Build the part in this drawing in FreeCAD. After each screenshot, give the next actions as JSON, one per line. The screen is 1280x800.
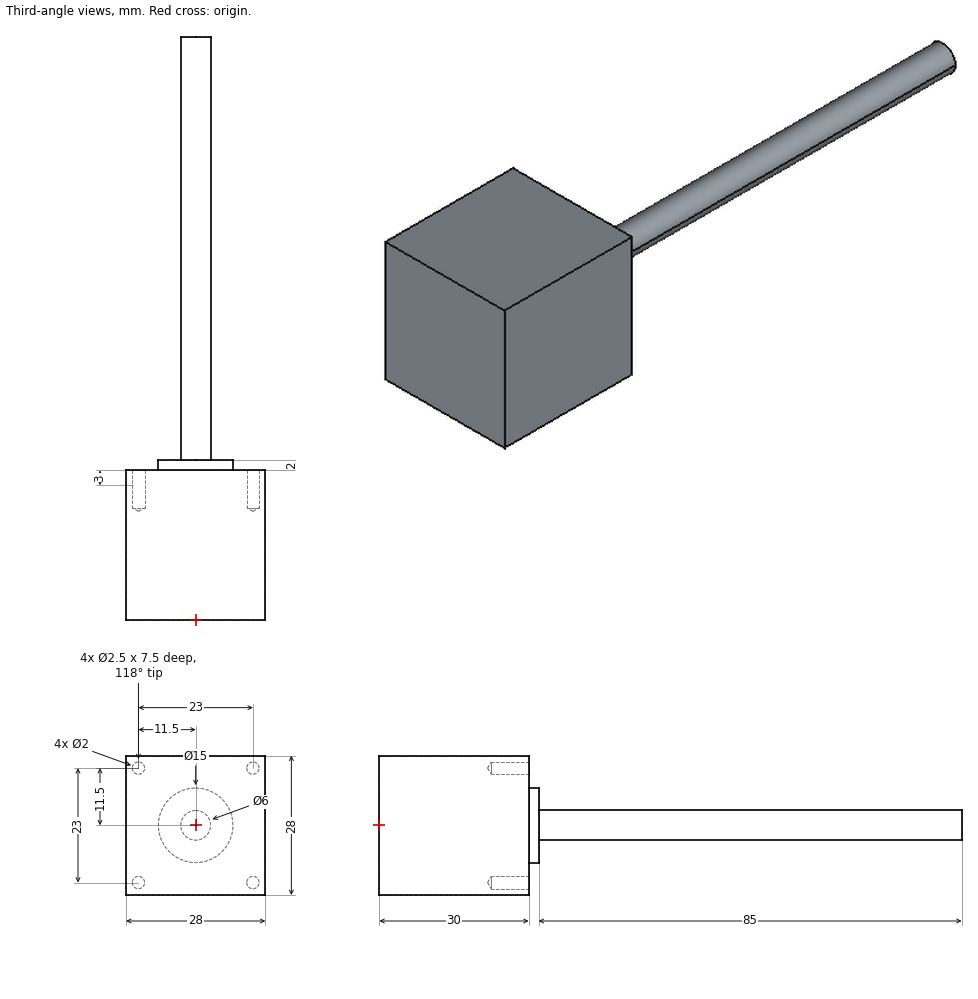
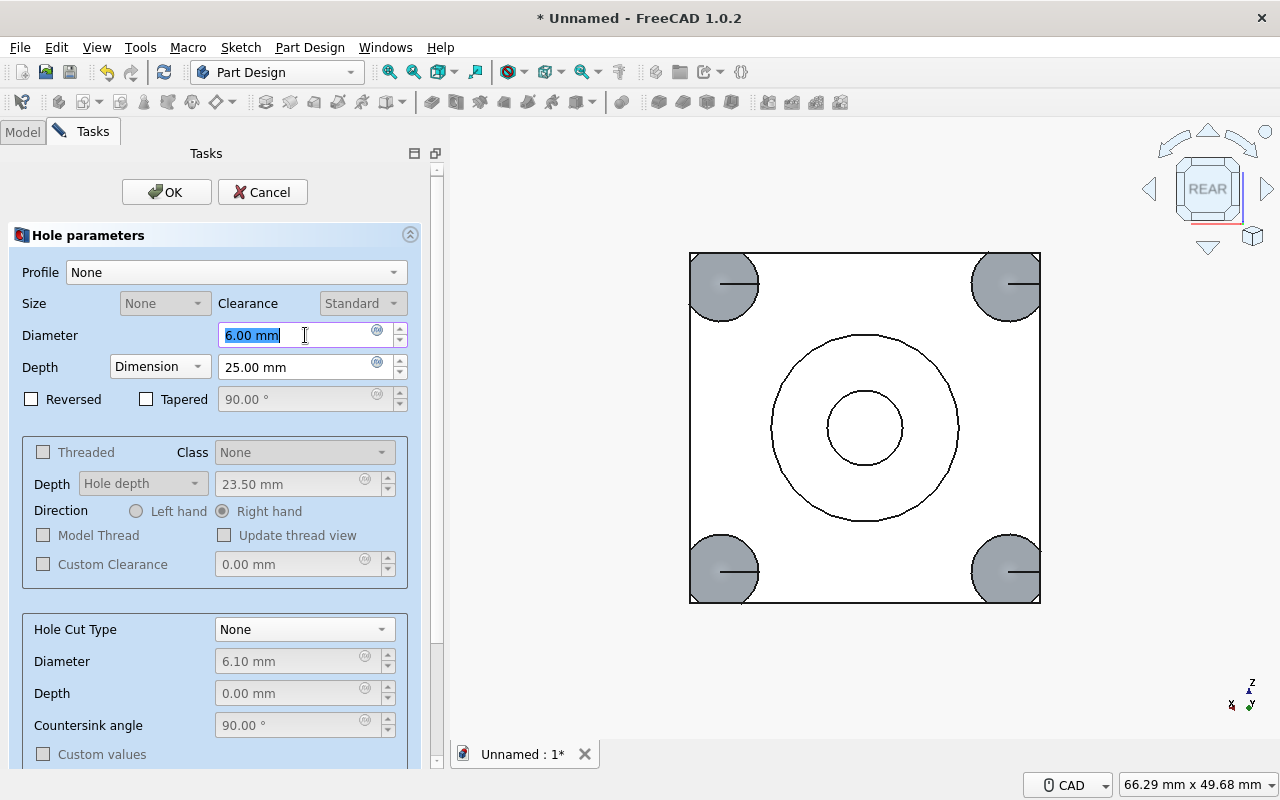
{"action": "type", "text": "2.5"}
{"action": "key", "text": "Tab"}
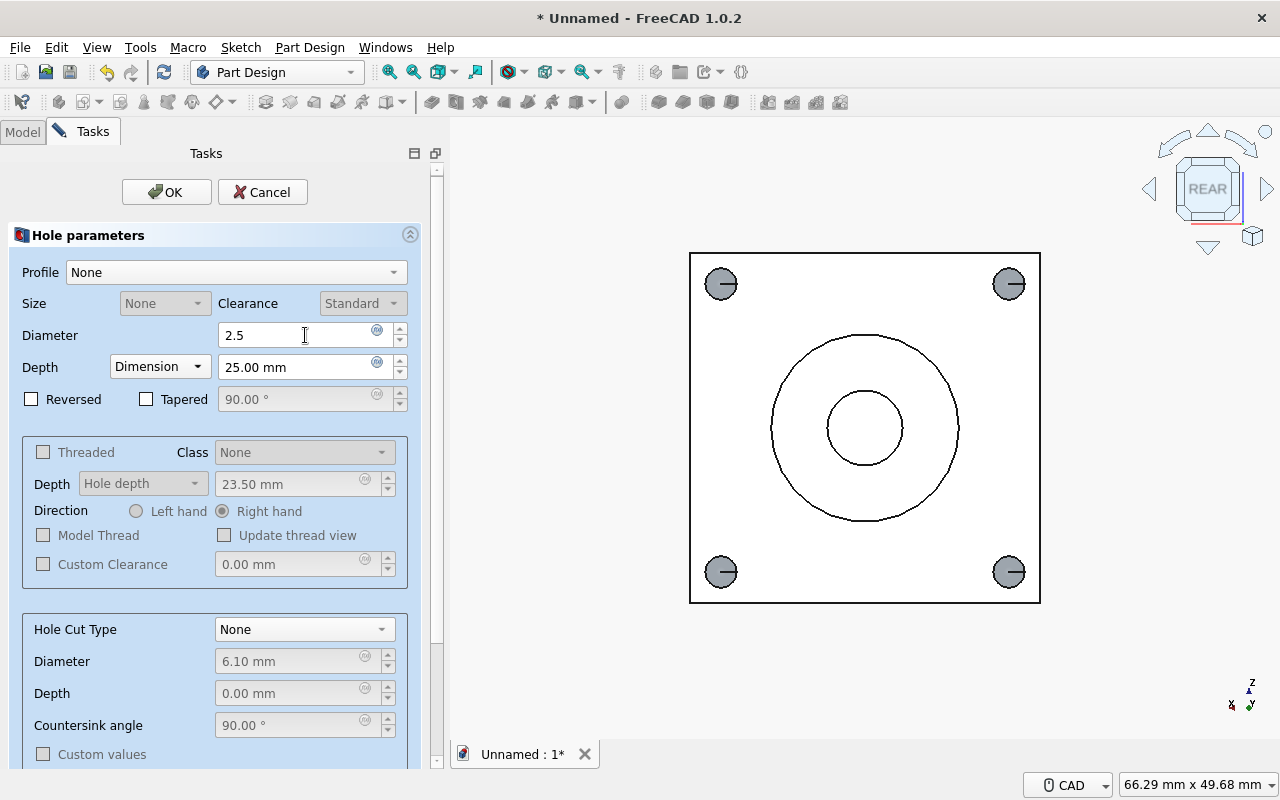
{"action": "triple_click", "coordinate": [305, 367]}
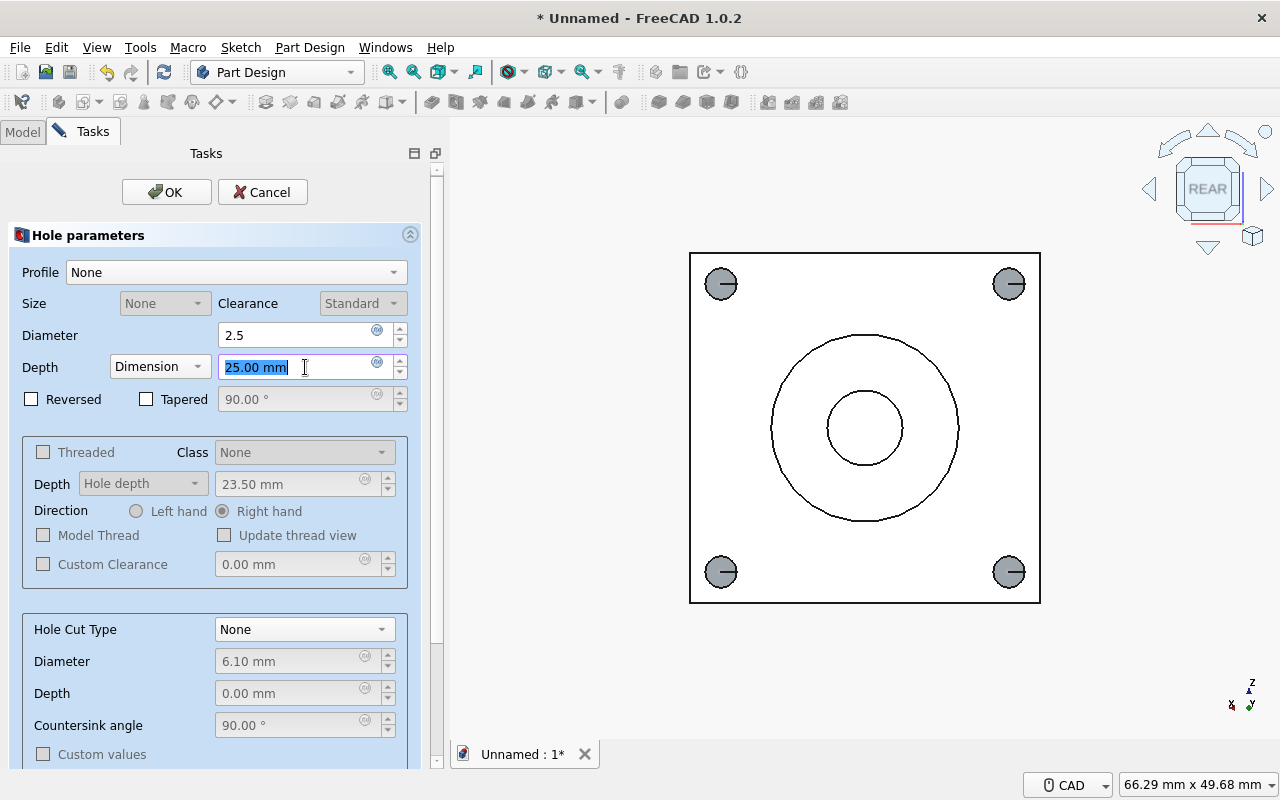
{"action": "type", "text": "7.5"}
{"action": "key", "text": "Tab"}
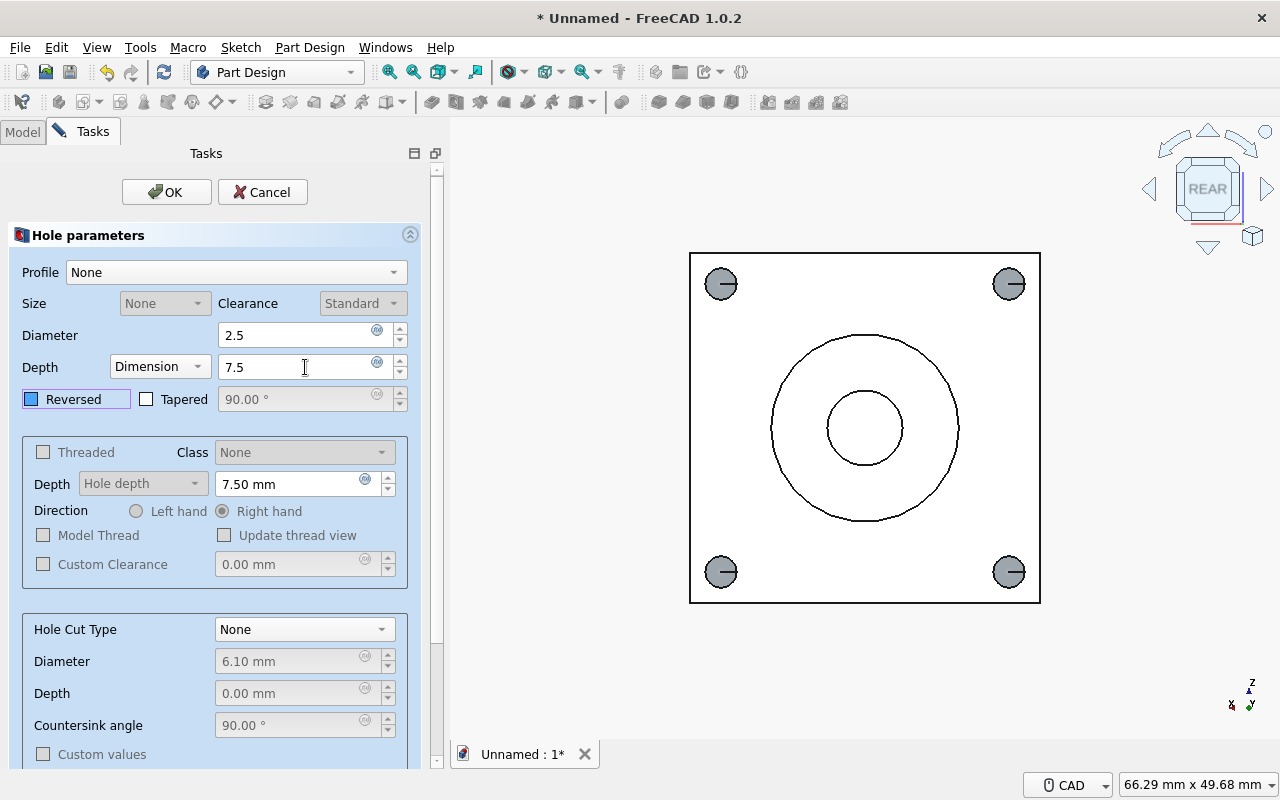
{"action": "left_click", "coordinate": [167, 192]}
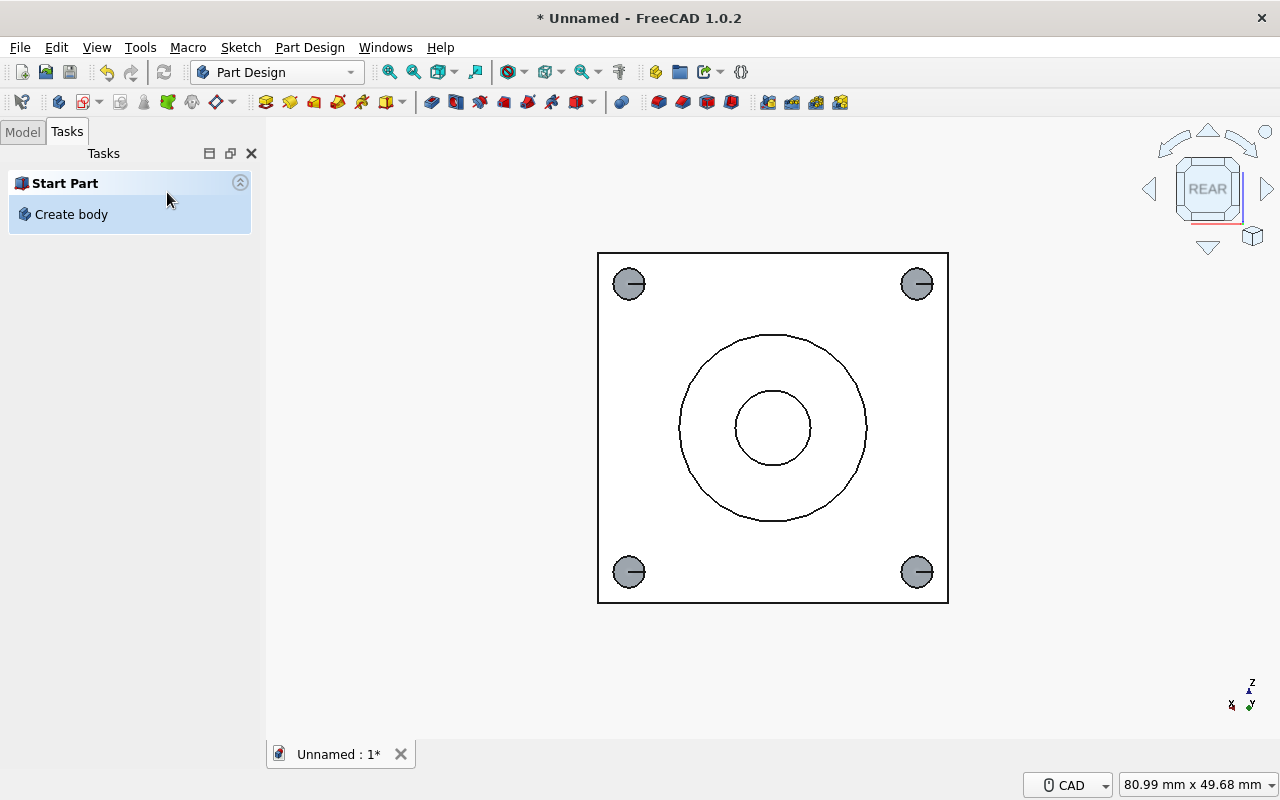
{"action": "key", "text": "0"}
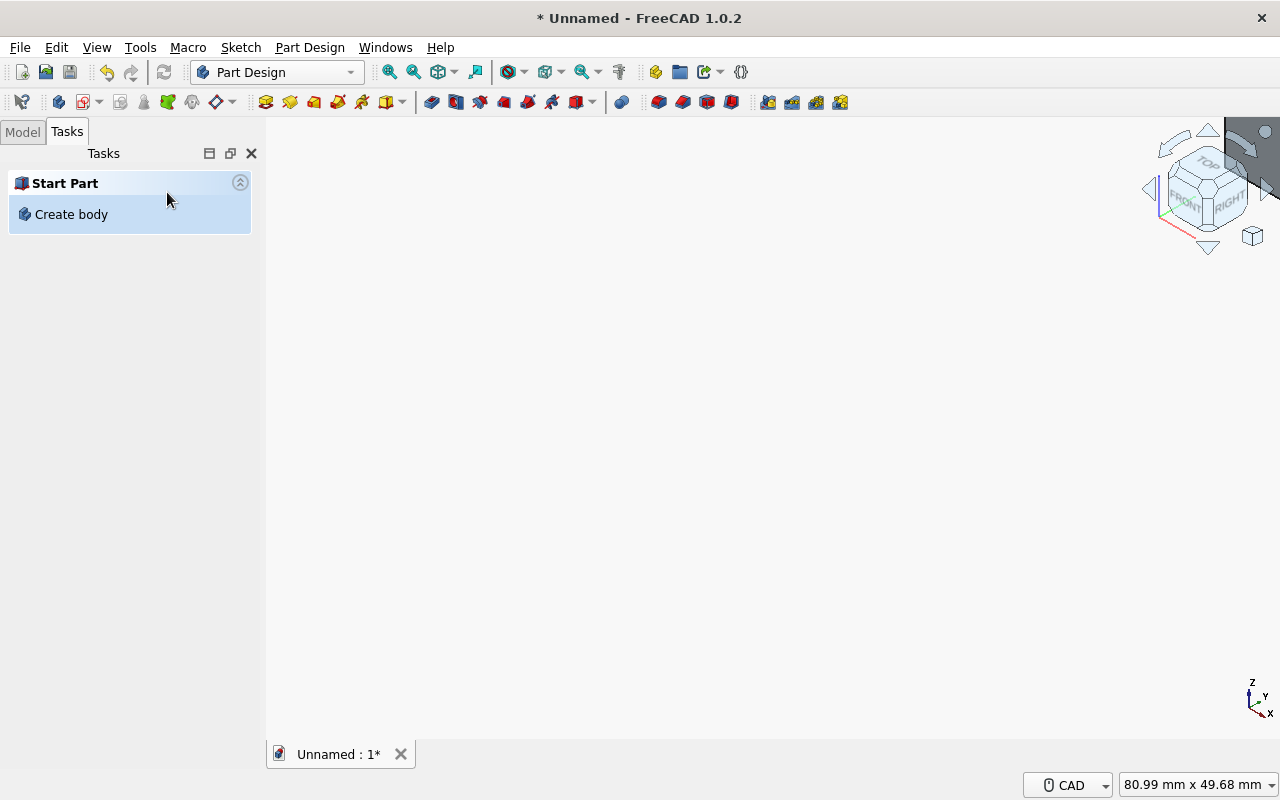
{"action": "left_click", "coordinate": [390, 72]}